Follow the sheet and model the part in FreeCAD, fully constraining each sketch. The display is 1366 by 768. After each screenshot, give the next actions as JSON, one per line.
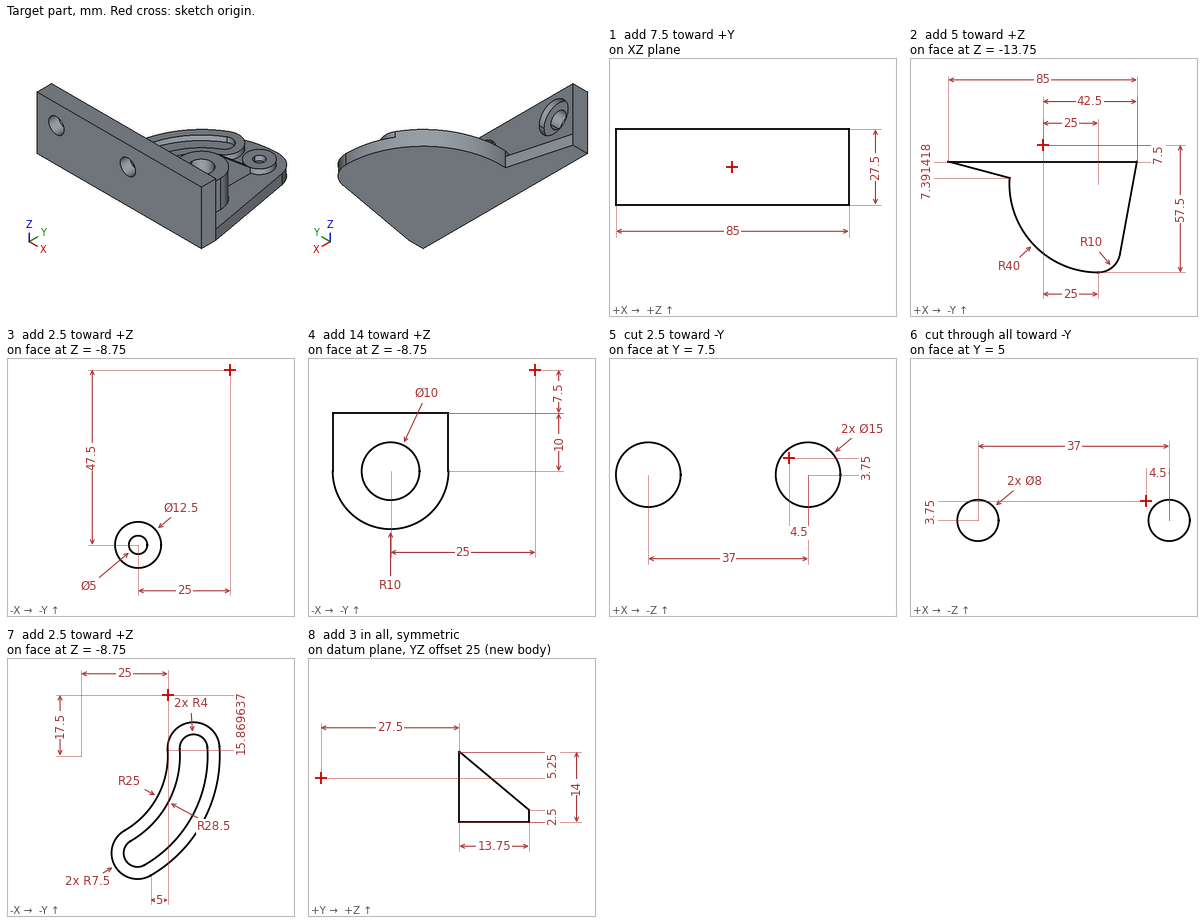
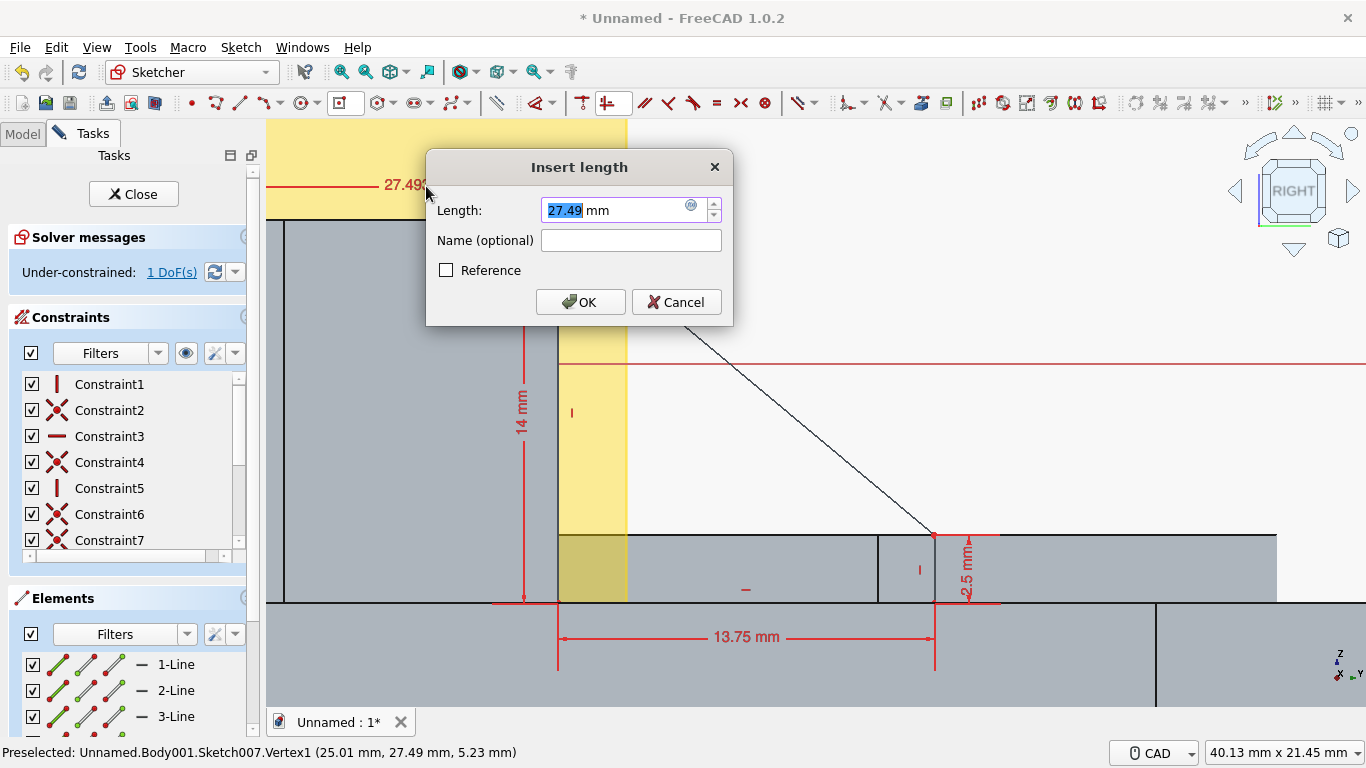
{"action": "type", "text": "27.5"}
{"action": "key", "text": "Return"}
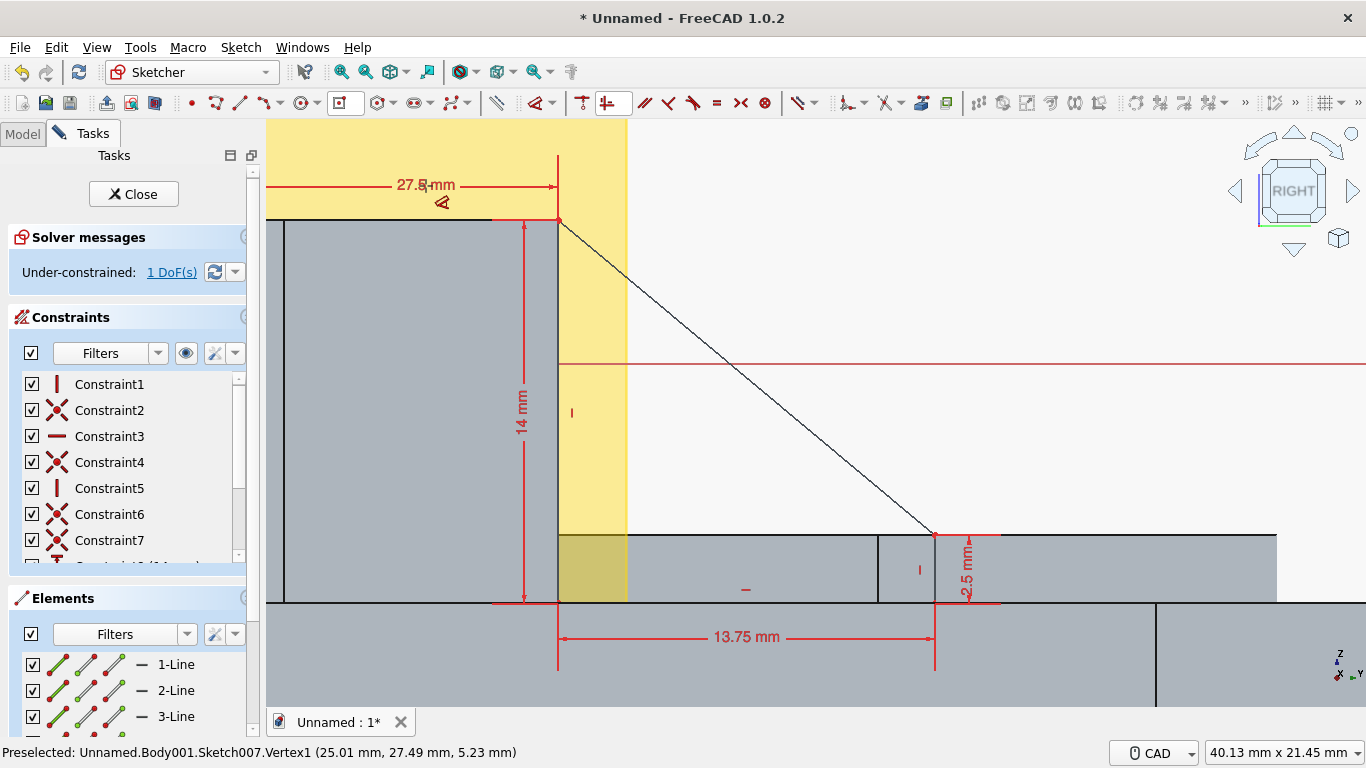
{"action": "left_click", "coordinate": [558, 220]}
{"action": "left_click", "coordinate": [592, 292]}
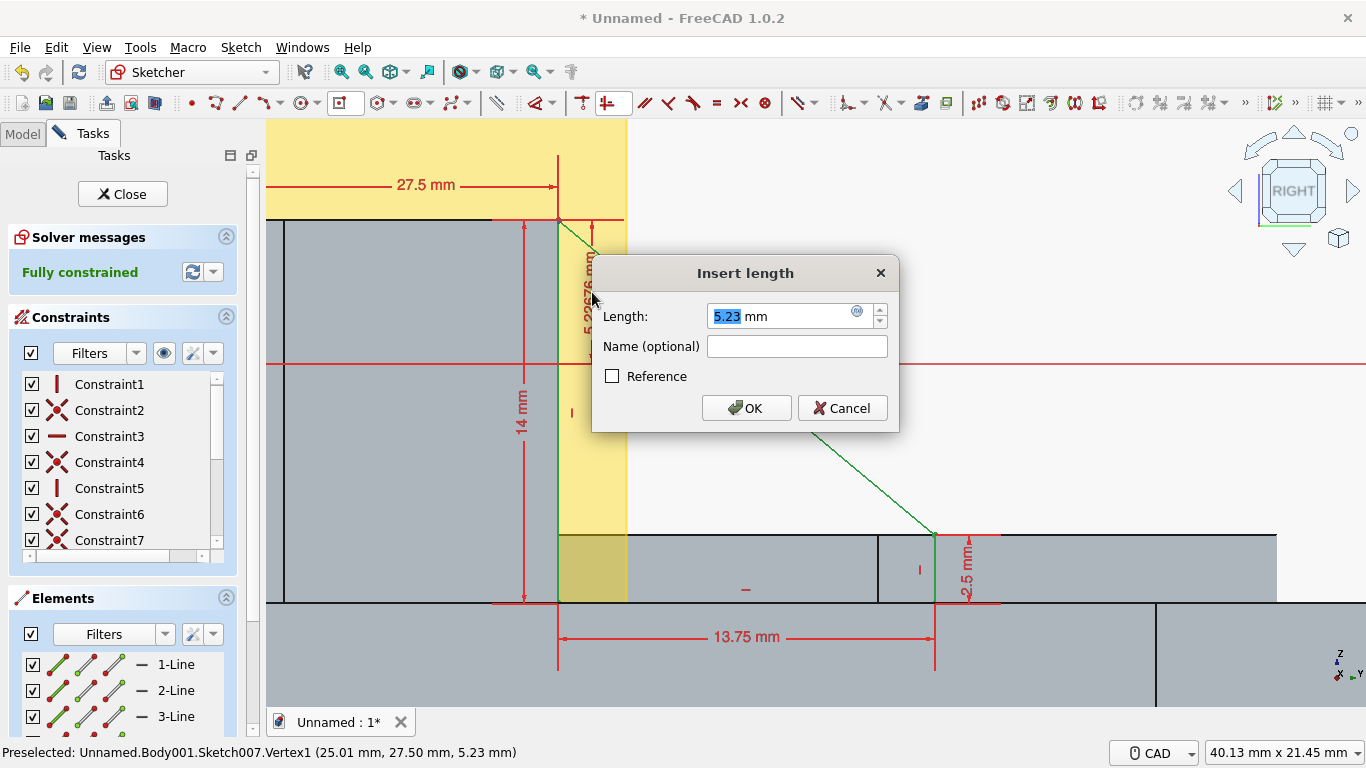
{"action": "type", "text": "5.25"}
{"action": "key", "text": "Return"}
{"action": "key", "text": "Escape"}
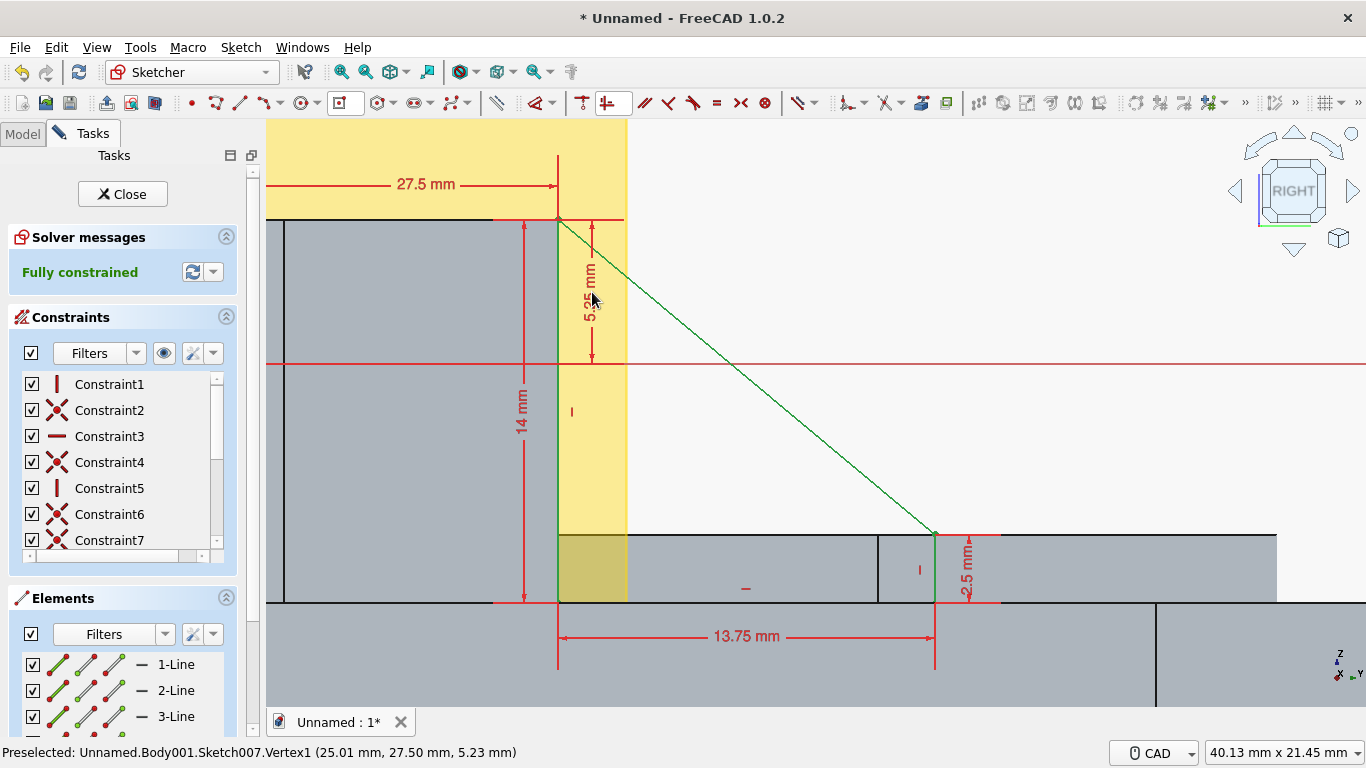
{"action": "left_click", "coordinate": [123, 194]}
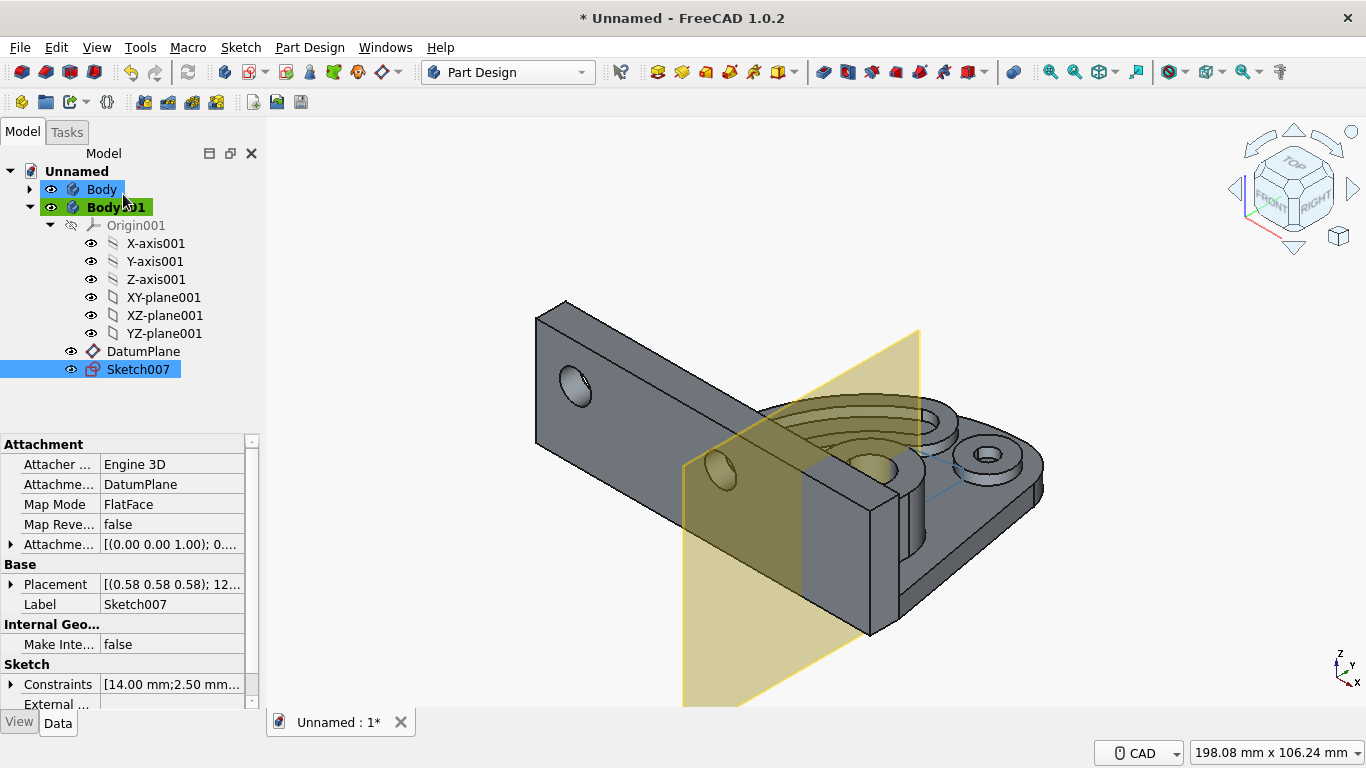
{"action": "left_click", "coordinate": [658, 72]}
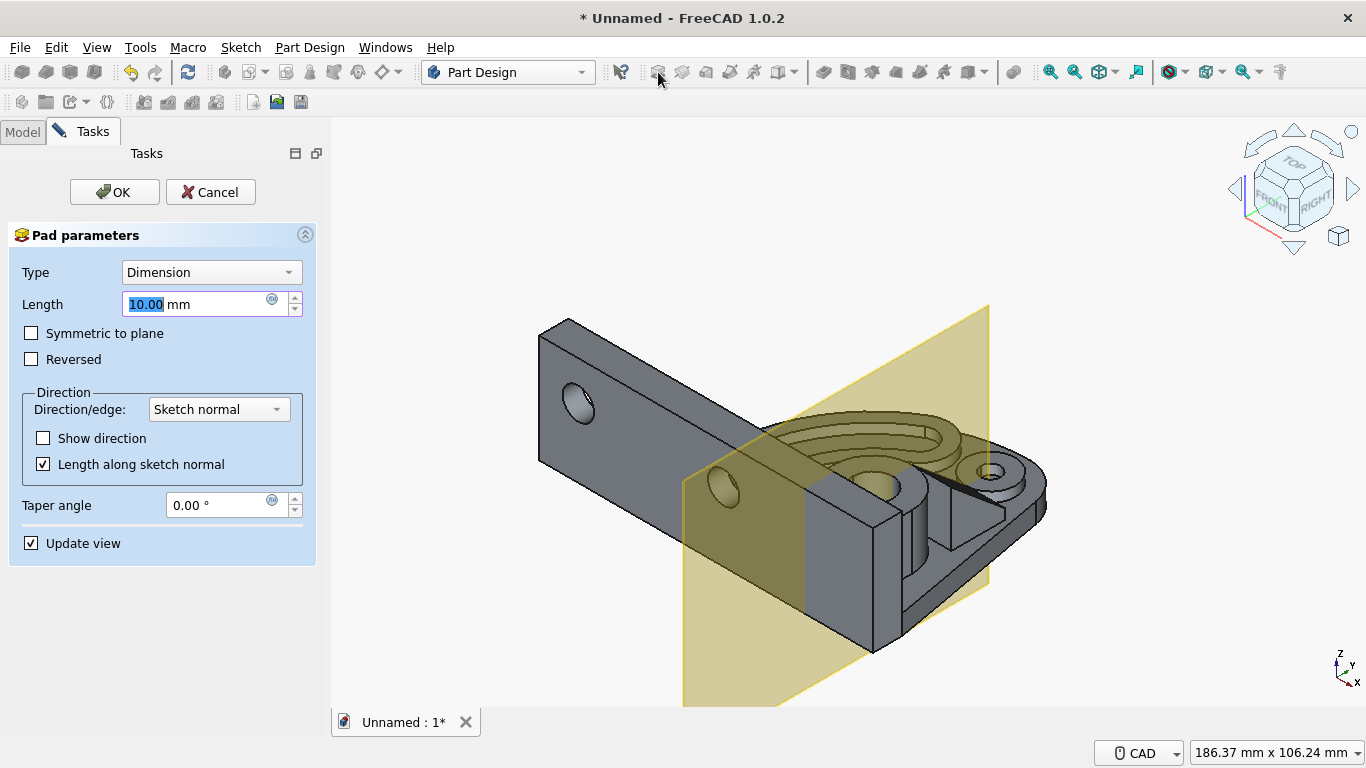
{"action": "type", "text": "3"}
{"action": "key", "text": "Tab"}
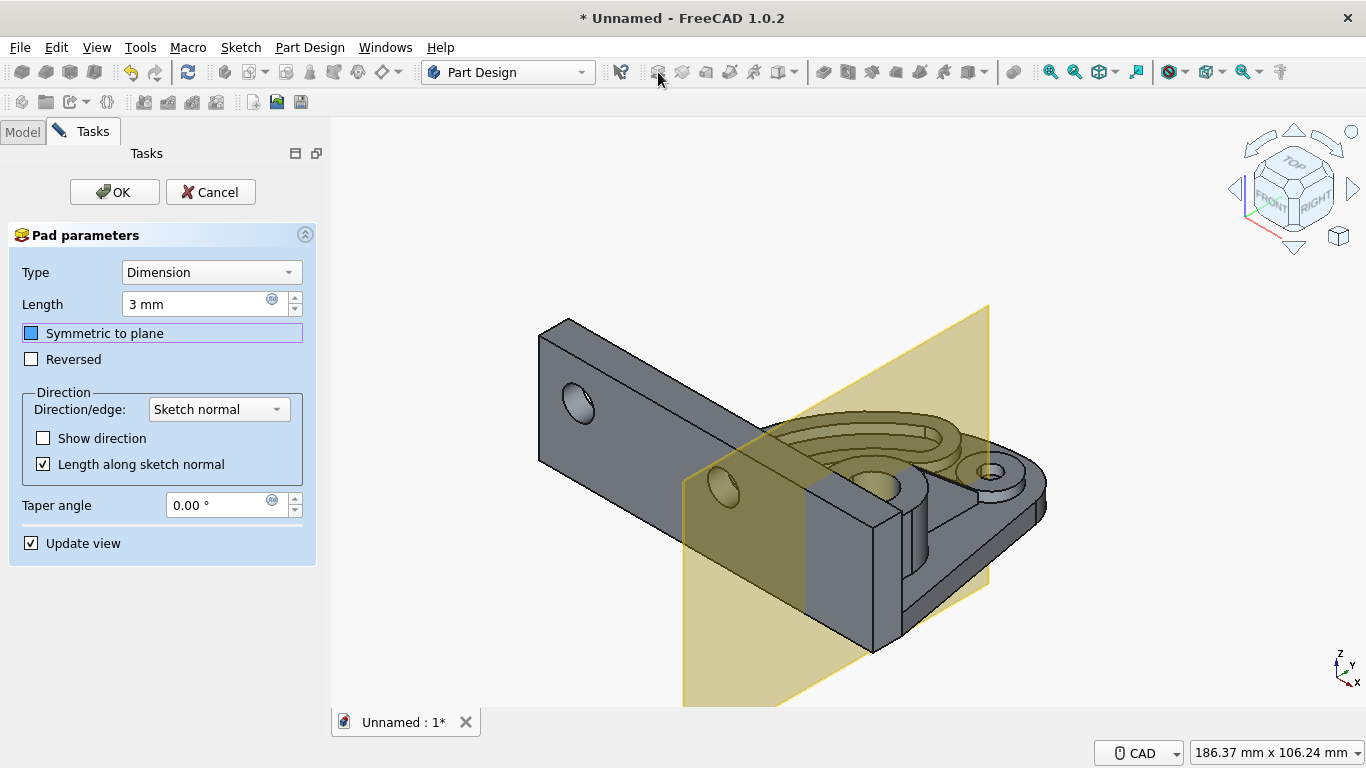
{"action": "left_click", "coordinate": [30, 333]}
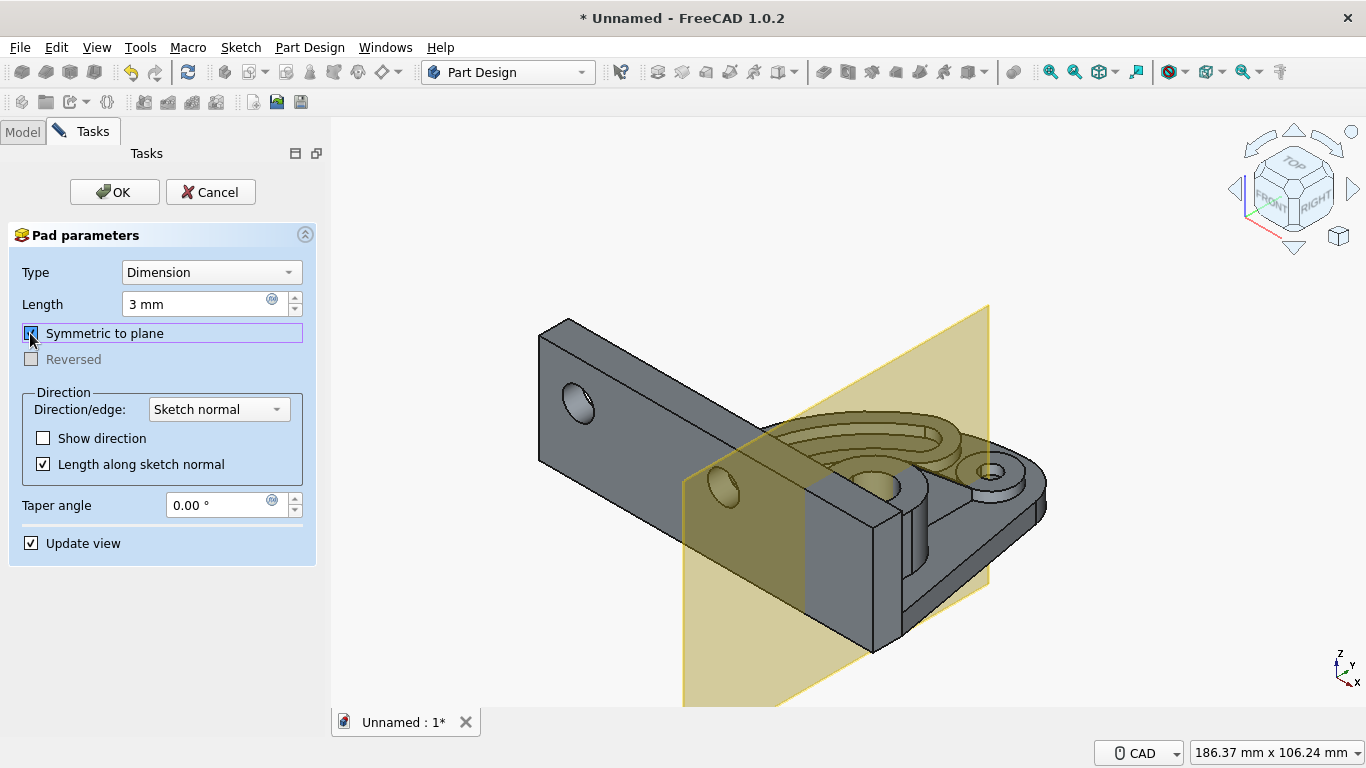
{"action": "left_click", "coordinate": [115, 192]}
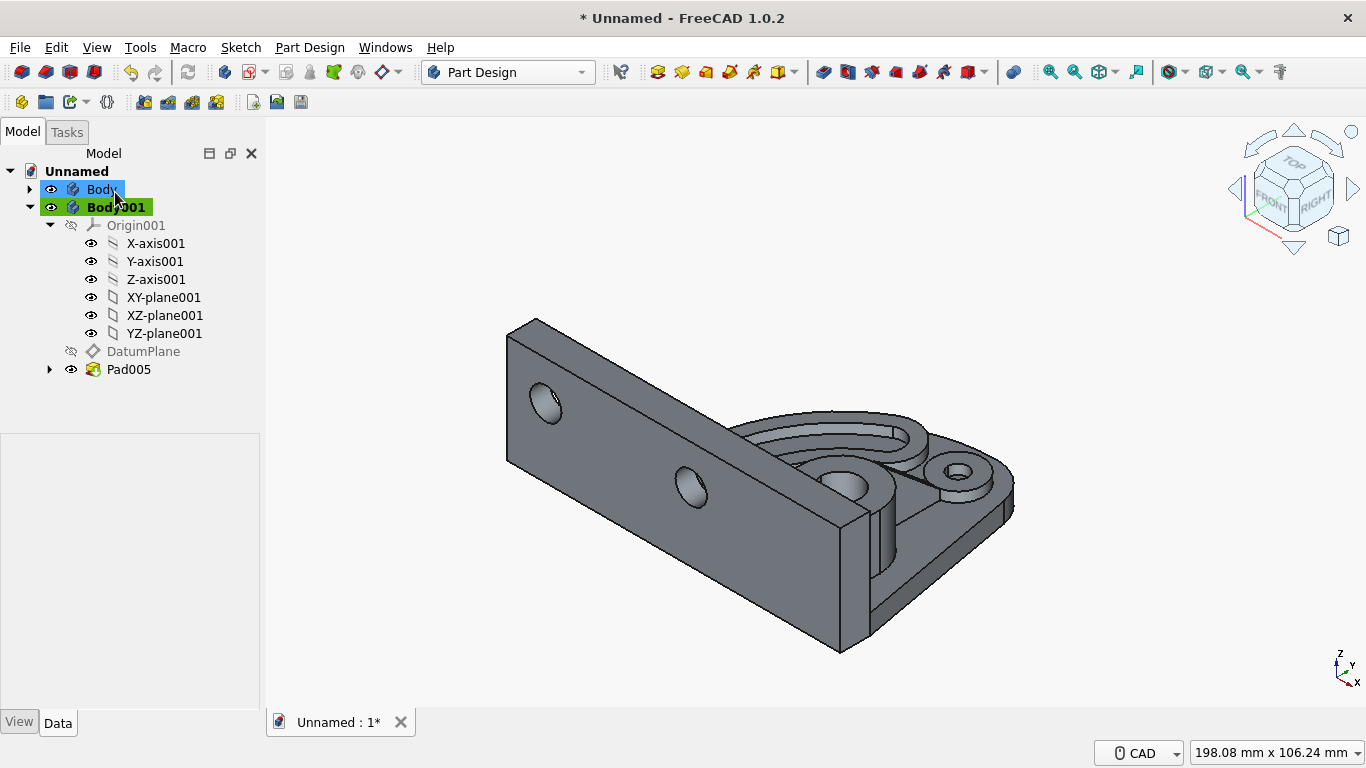
{"action": "left_click", "coordinate": [1052, 72]}